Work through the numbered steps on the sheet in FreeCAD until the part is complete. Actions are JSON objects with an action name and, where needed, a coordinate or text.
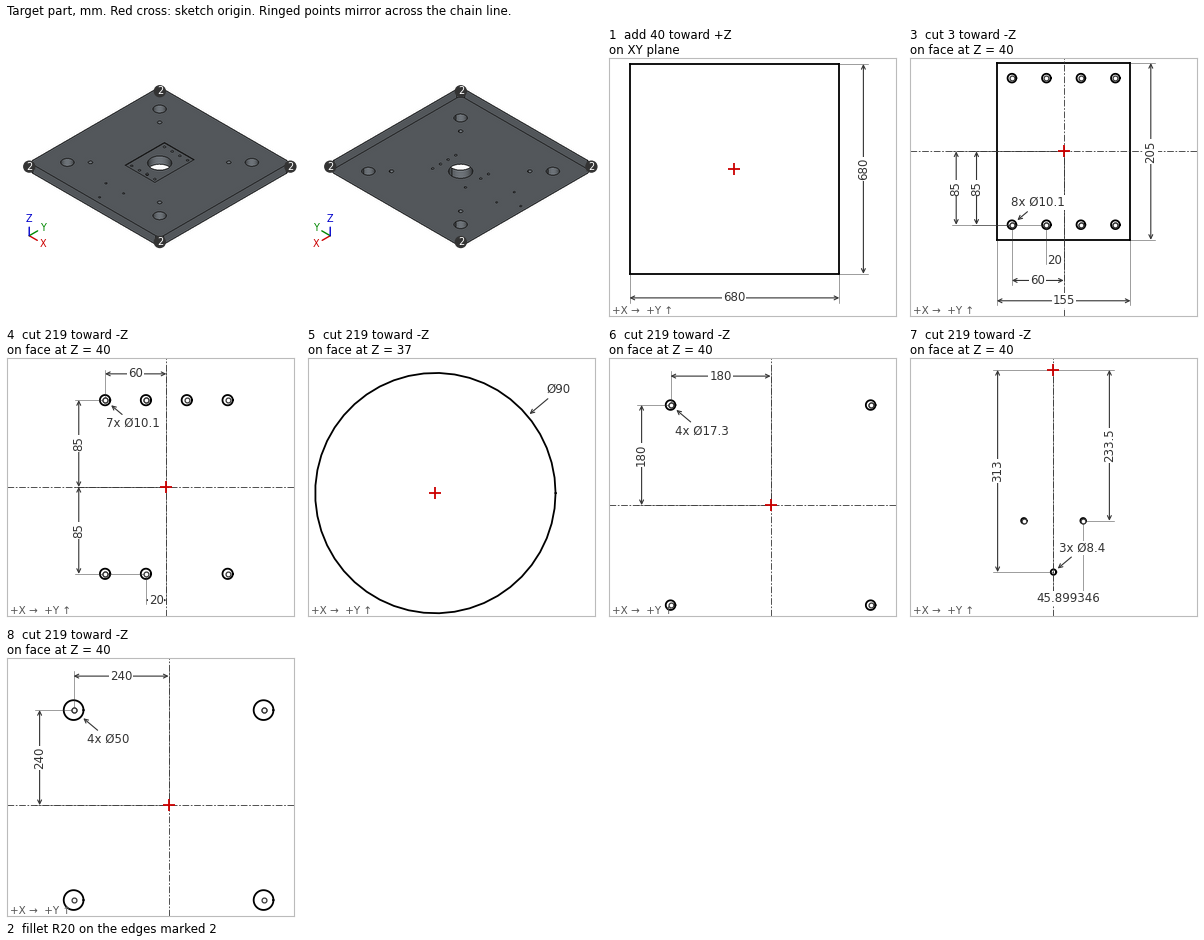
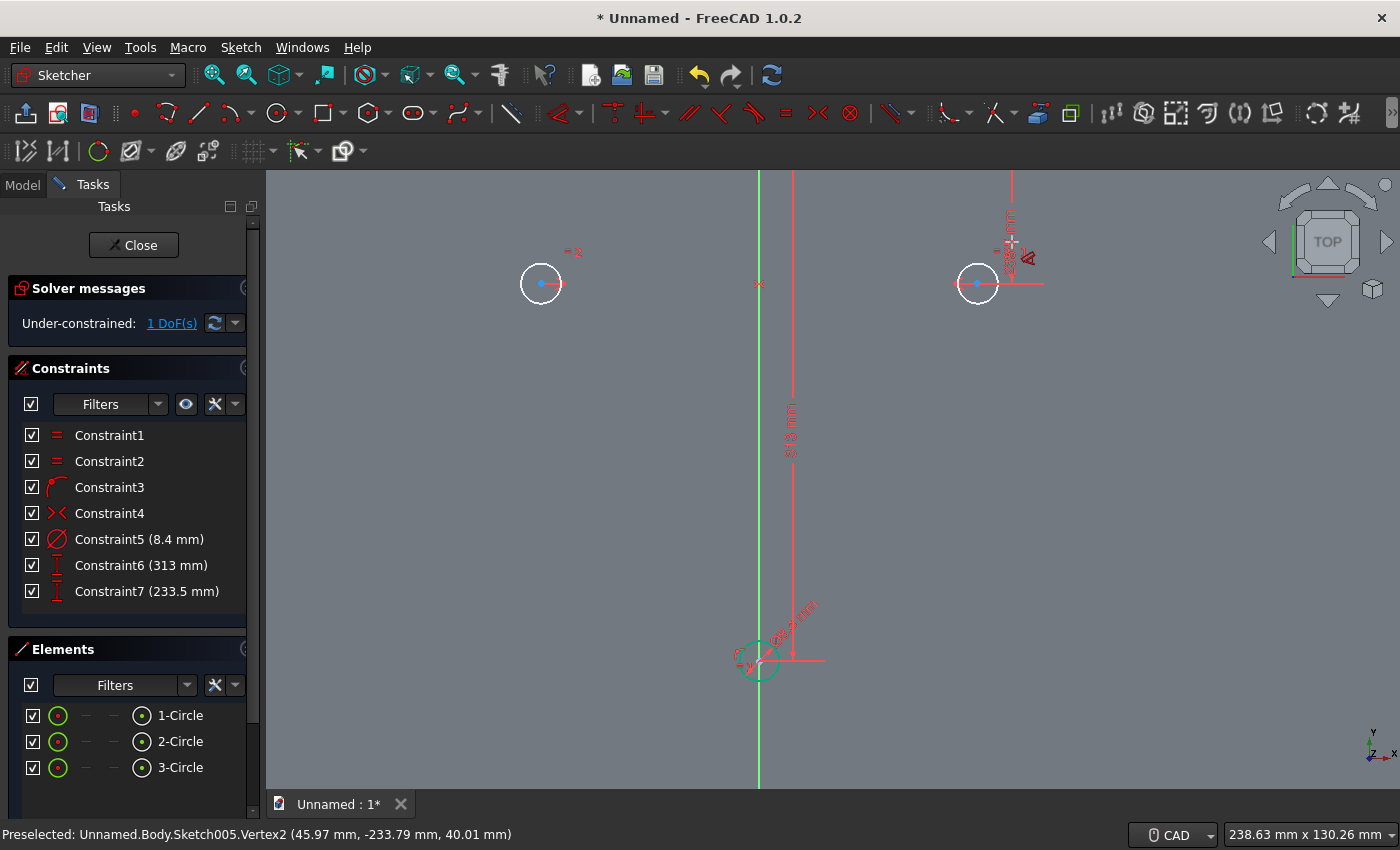
{"action": "left_click", "coordinate": [978, 284]}
{"action": "left_click", "coordinate": [869, 318]}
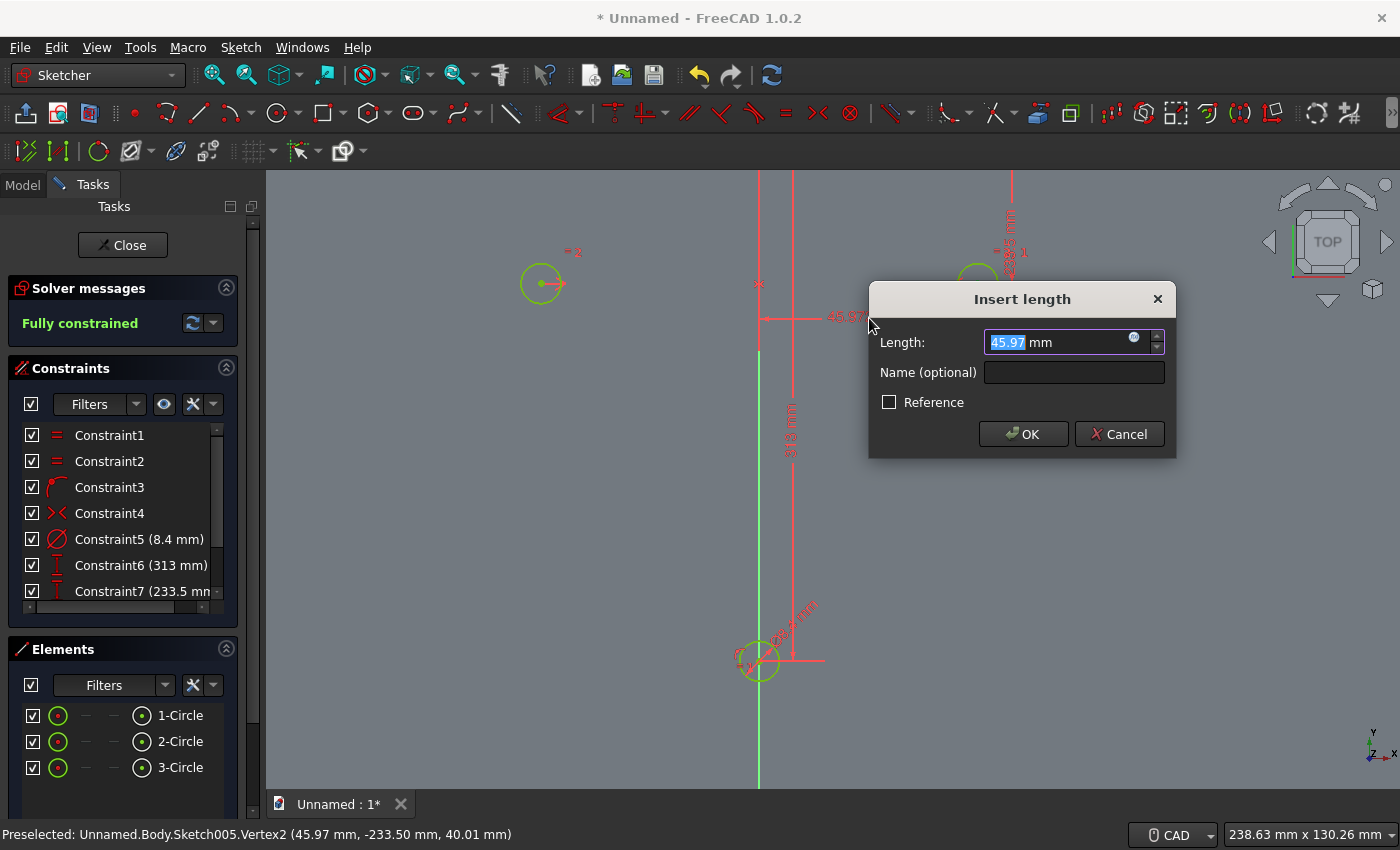
{"action": "type", "text": "45.899346"}
{"action": "key", "text": "Return"}
{"action": "key", "text": "Escape"}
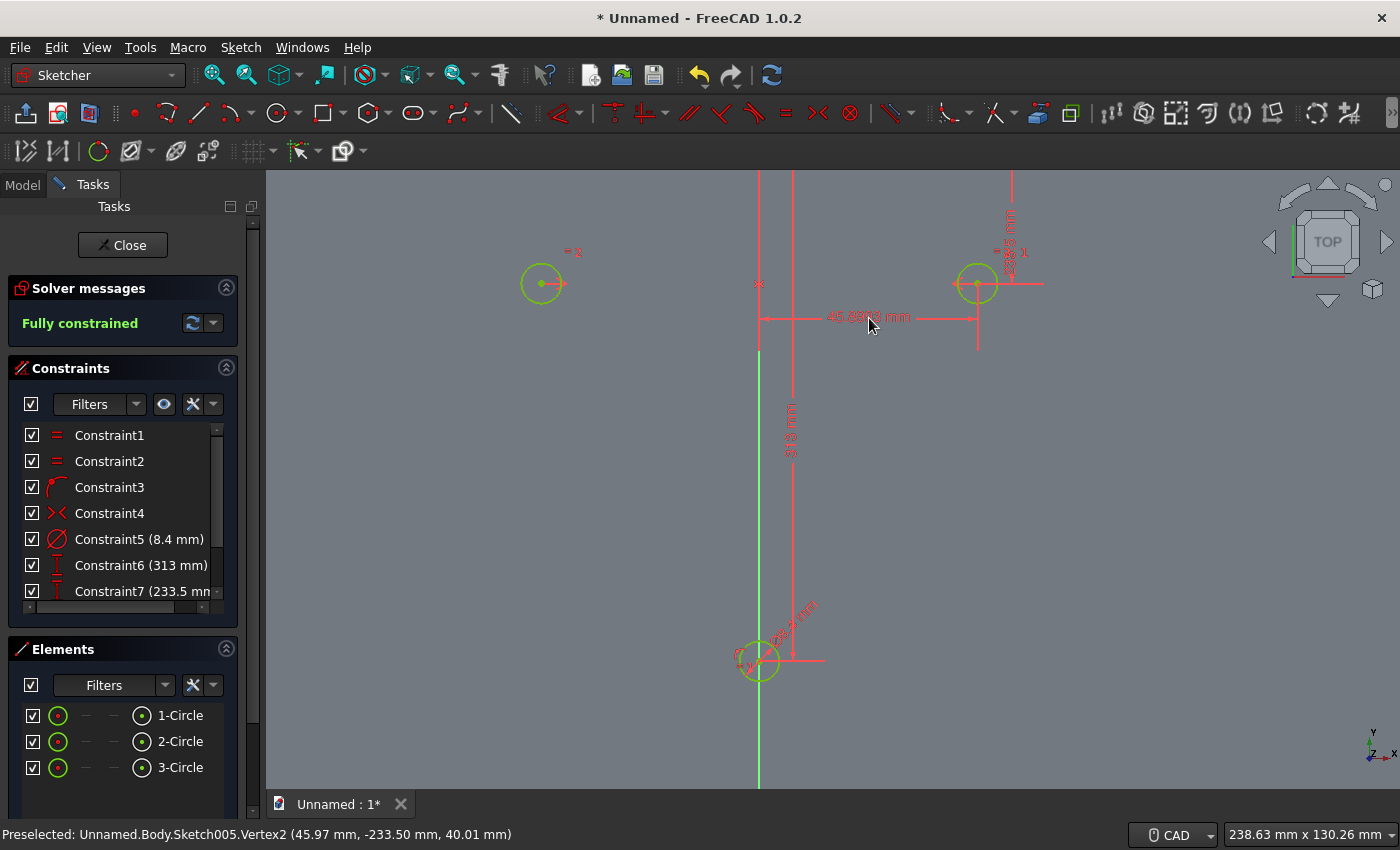
{"action": "left_click", "coordinate": [123, 245]}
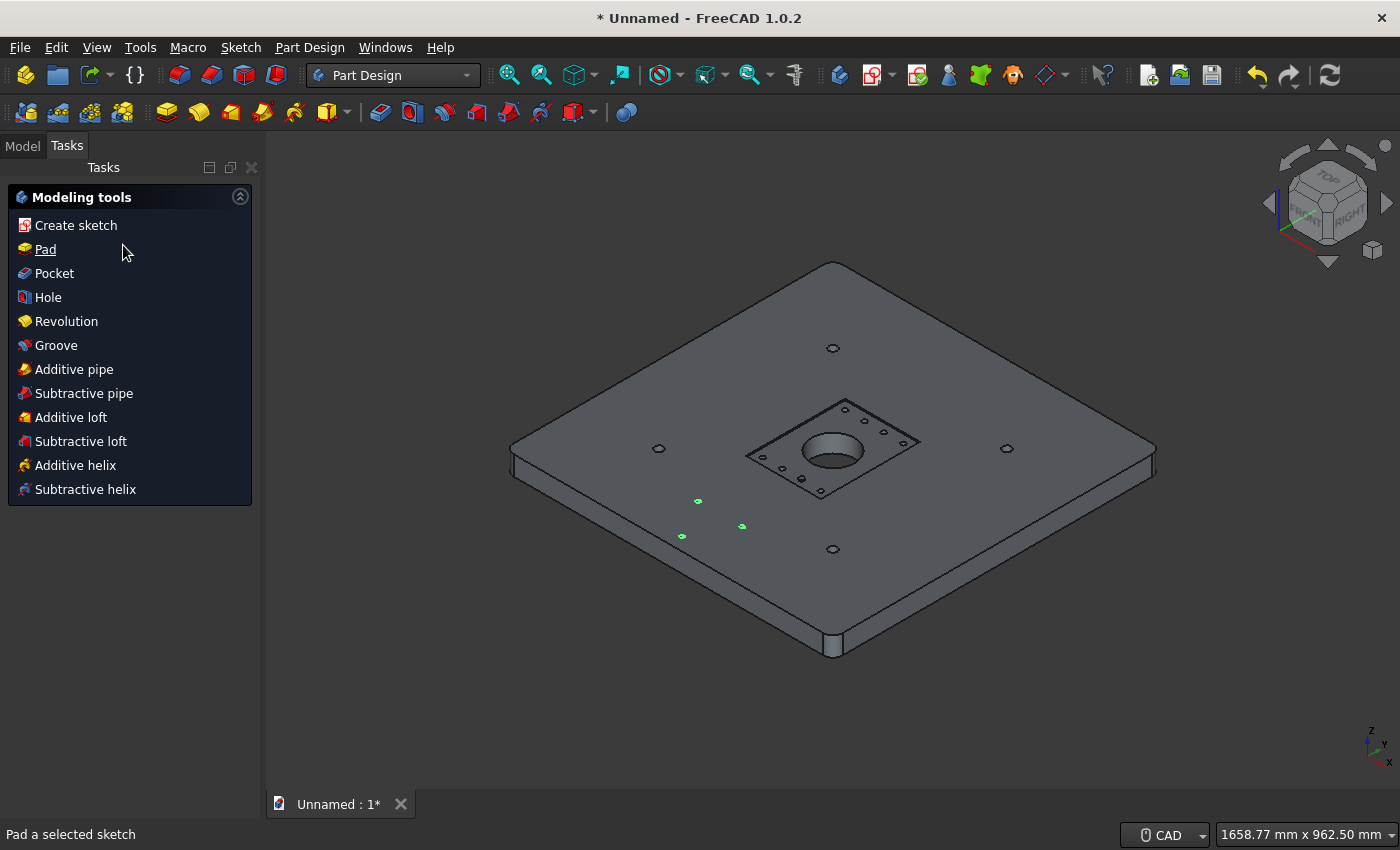
{"action": "left_click", "coordinate": [382, 112]}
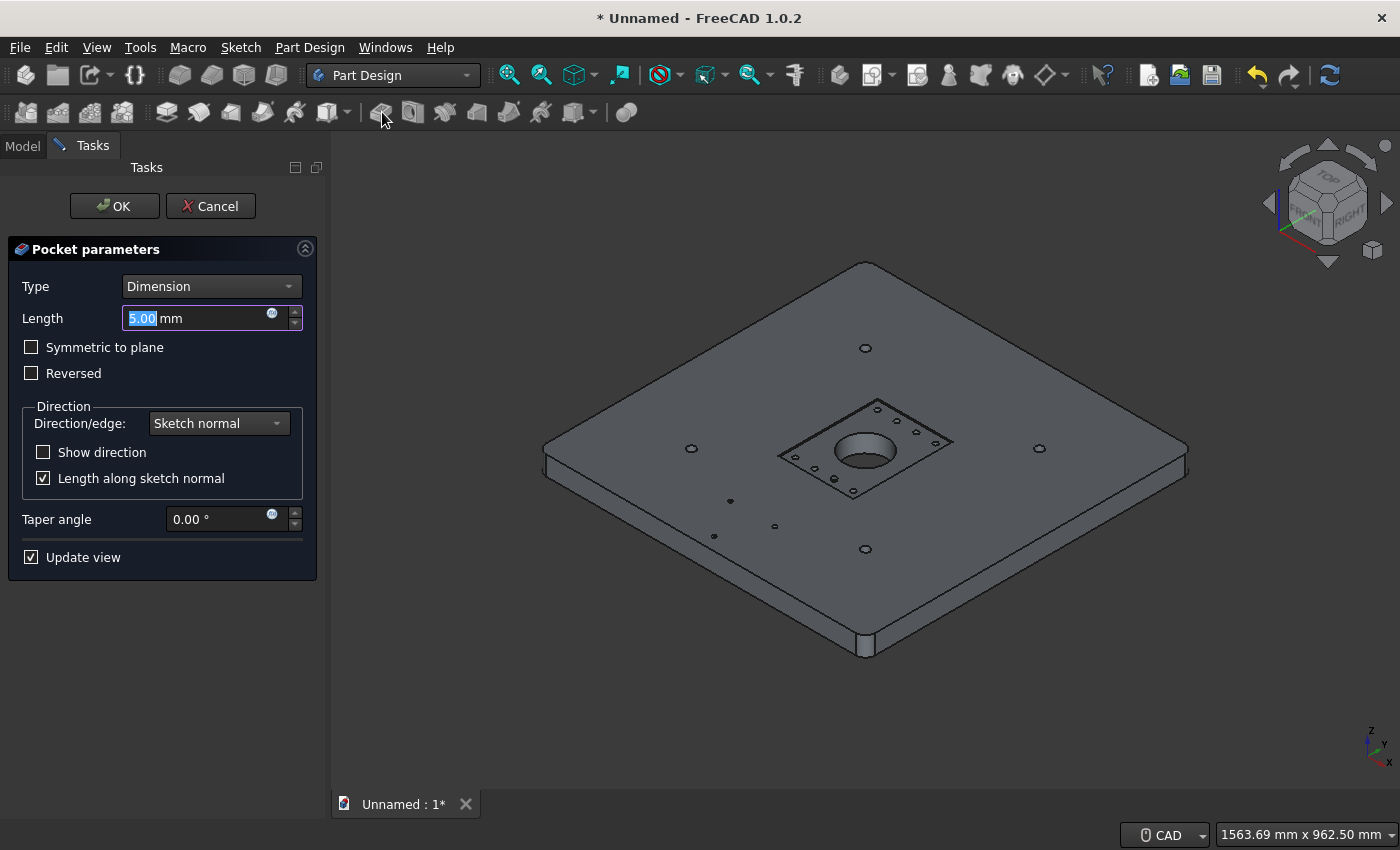
{"action": "type", "text": "219"}
{"action": "key", "text": "Tab"}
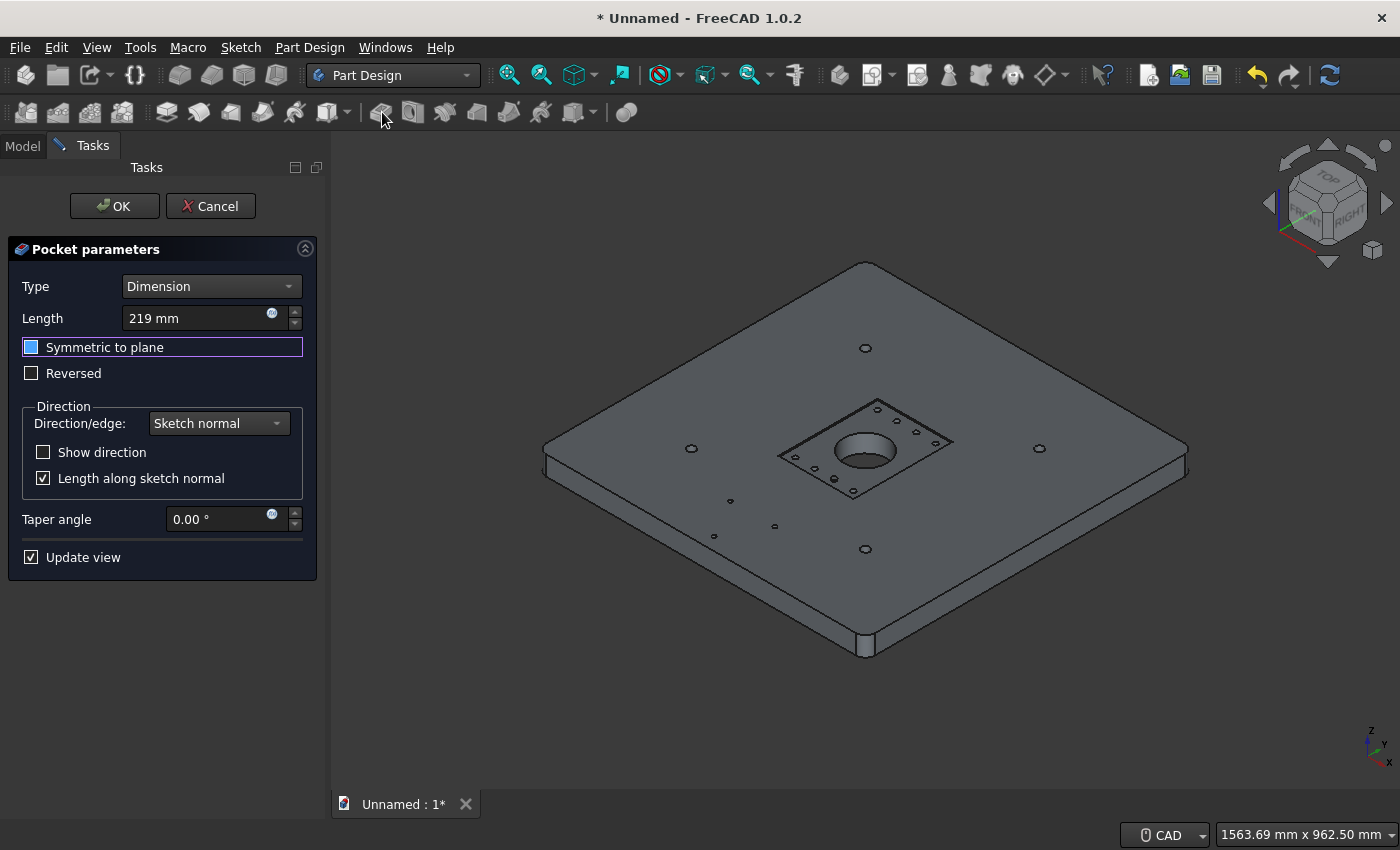
{"action": "left_click", "coordinate": [115, 206]}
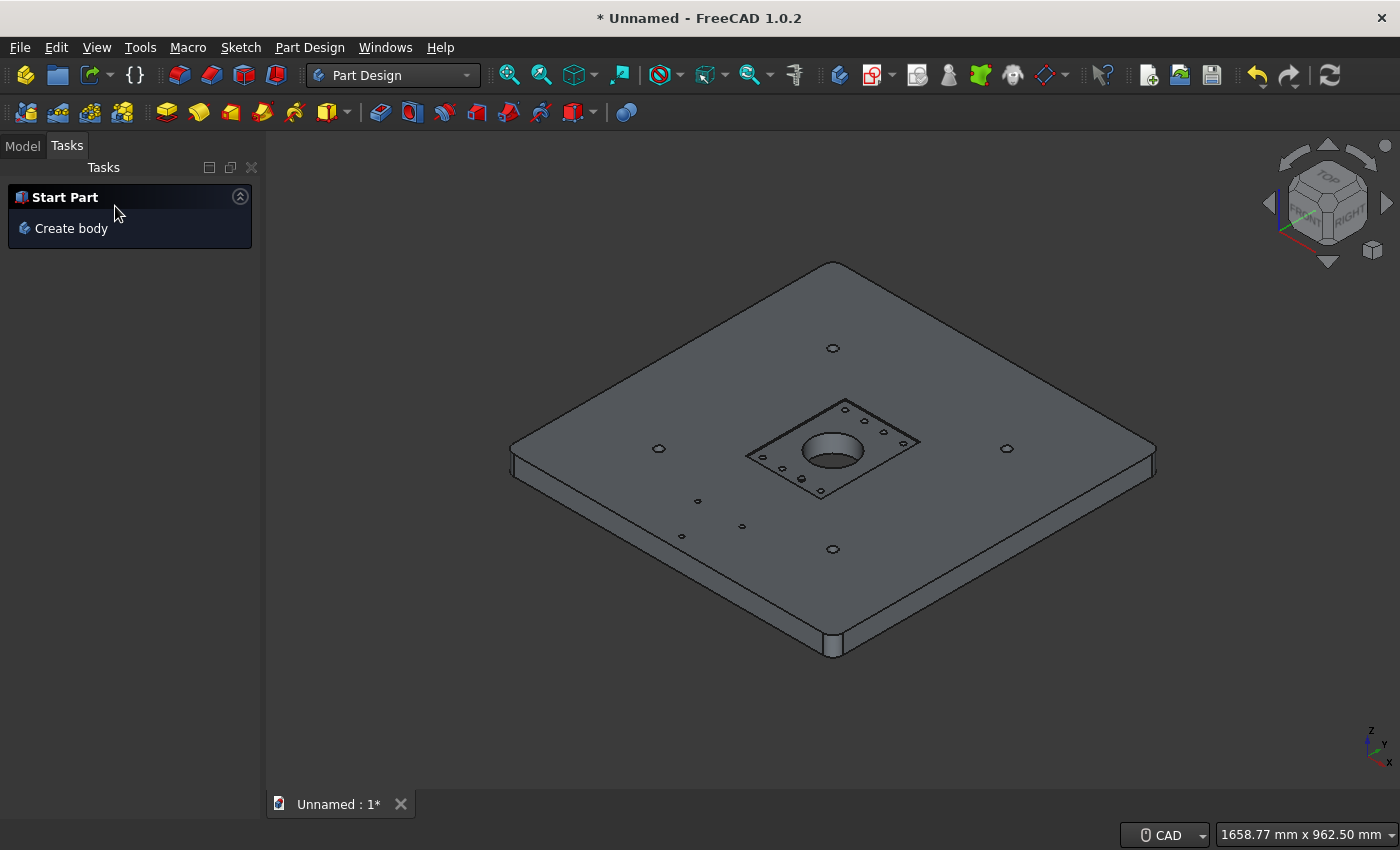
{"action": "left_click", "coordinate": [927, 502]}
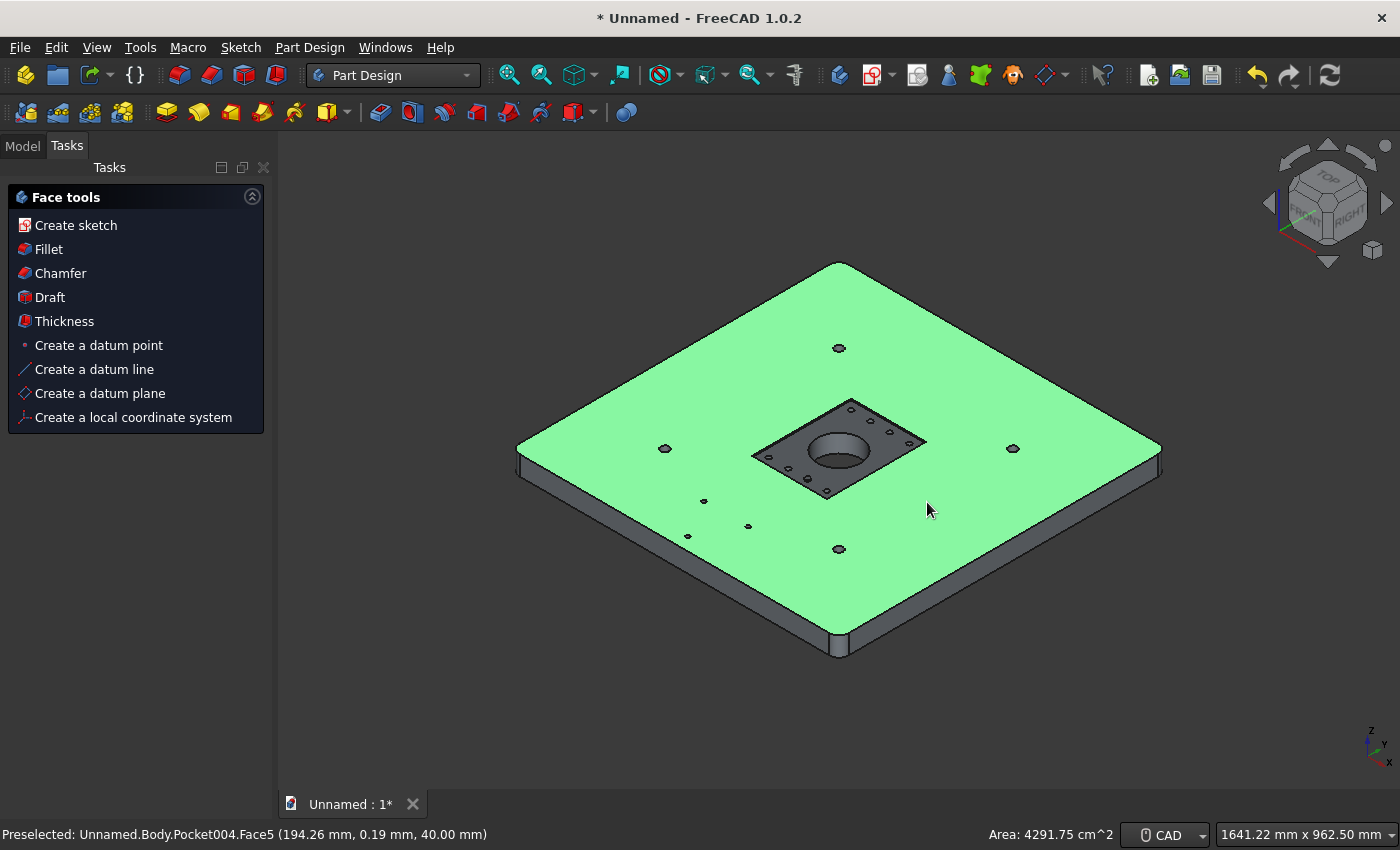
{"action": "left_click", "coordinate": [872, 76]}